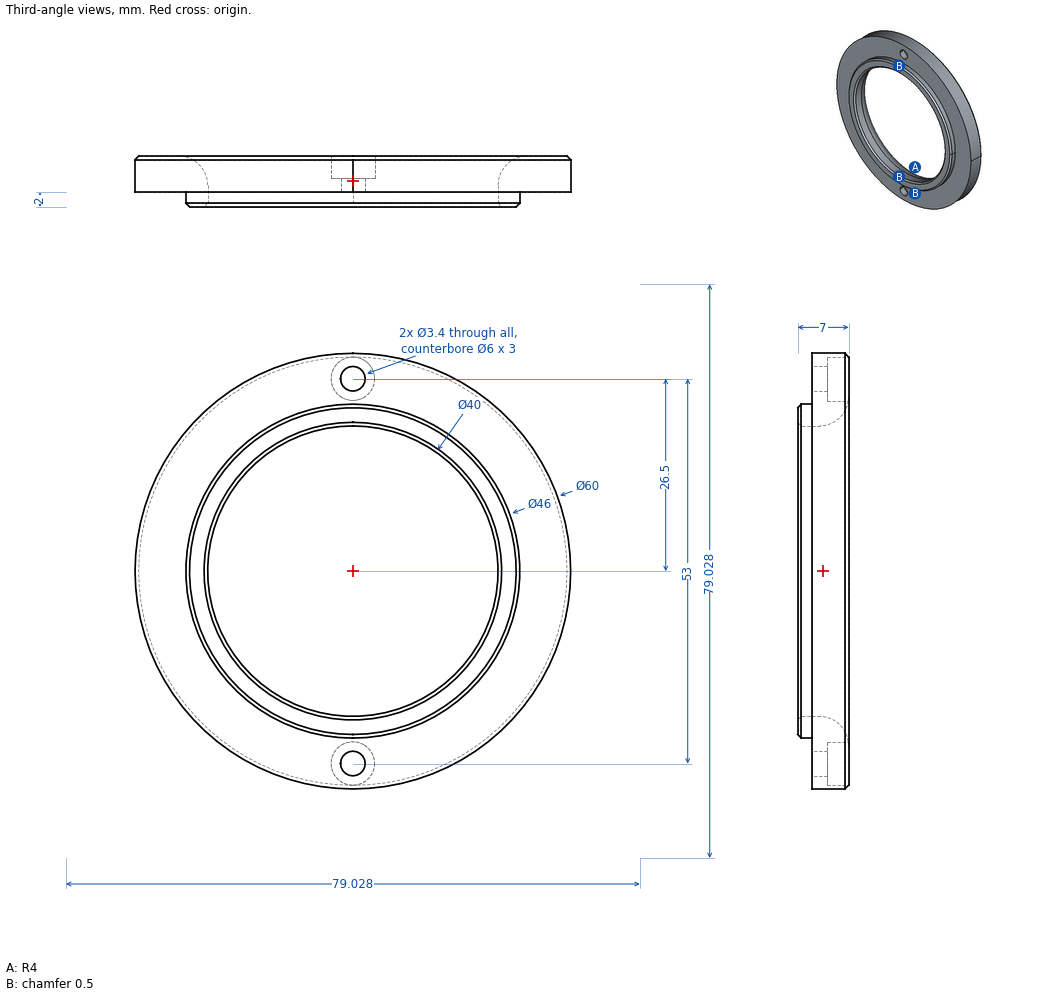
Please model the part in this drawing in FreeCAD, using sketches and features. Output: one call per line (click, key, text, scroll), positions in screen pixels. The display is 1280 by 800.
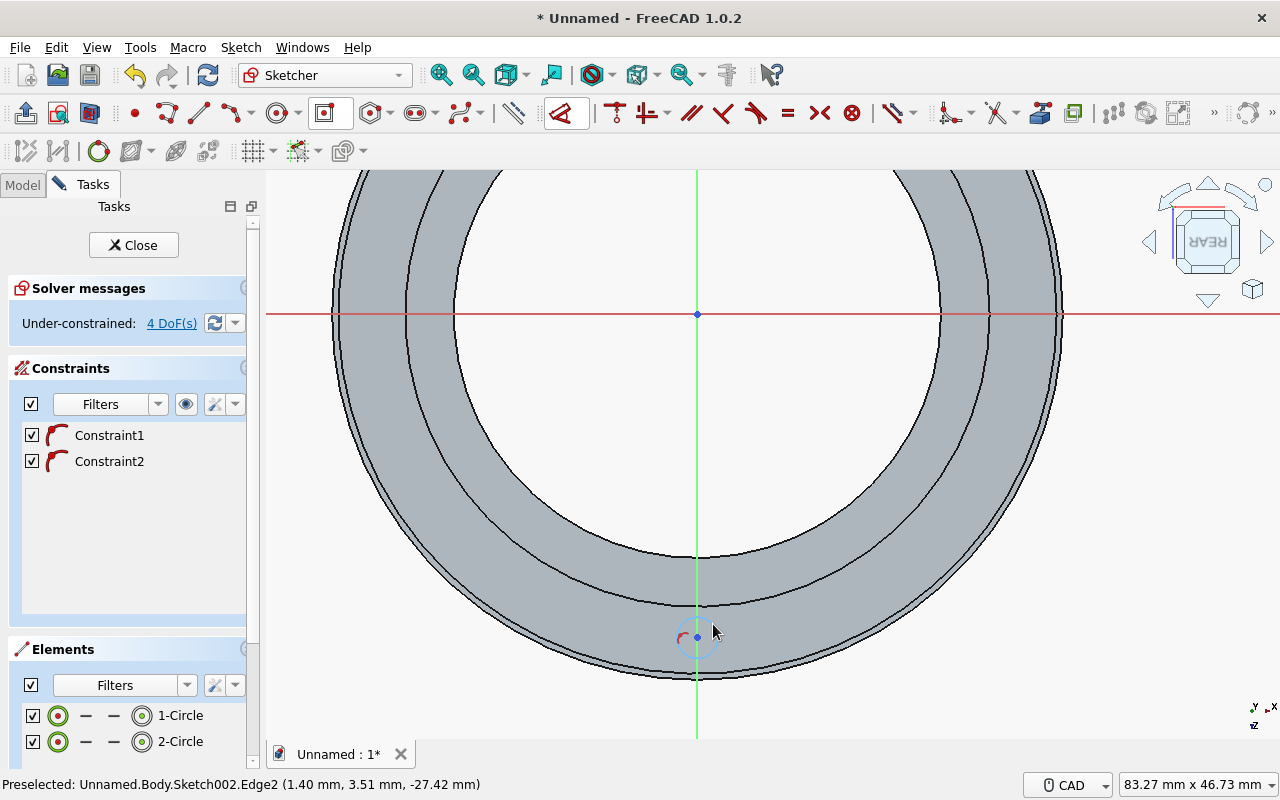
click(712, 623)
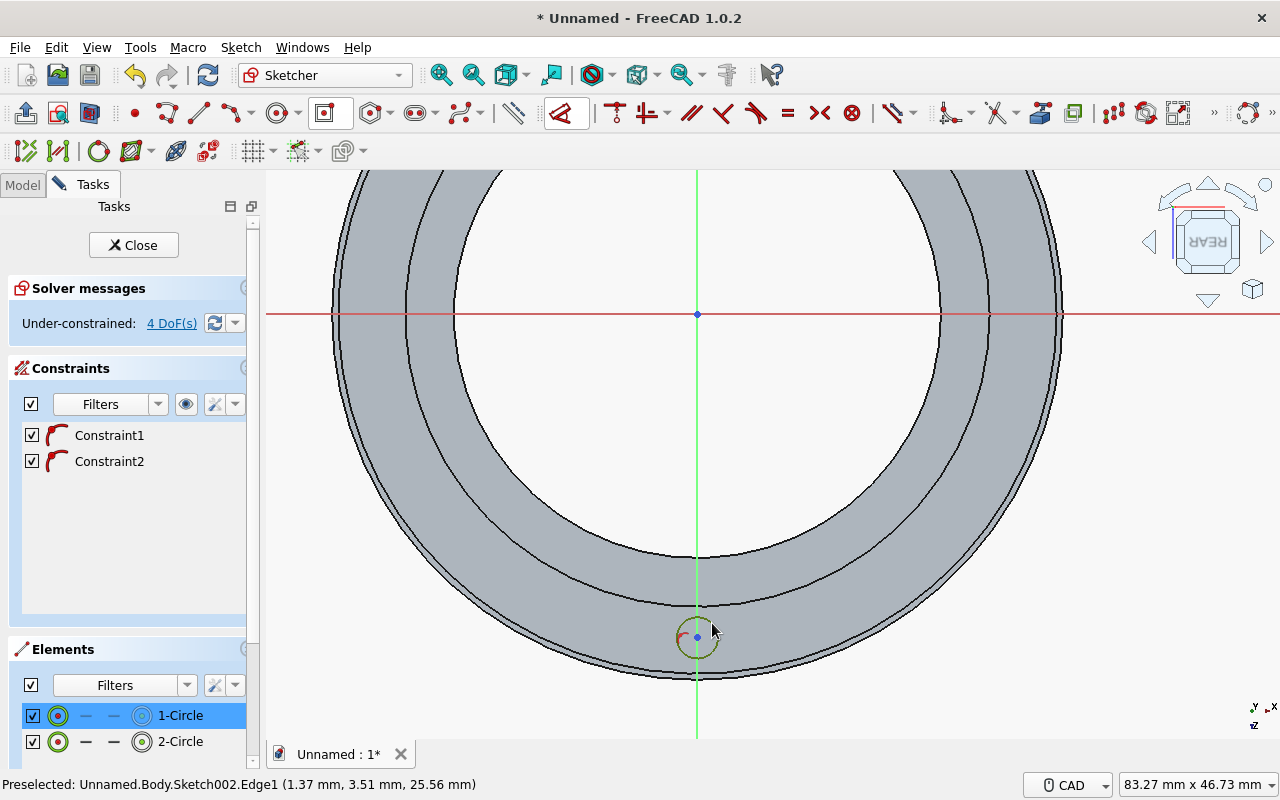
scroll(713, 625, down, 3)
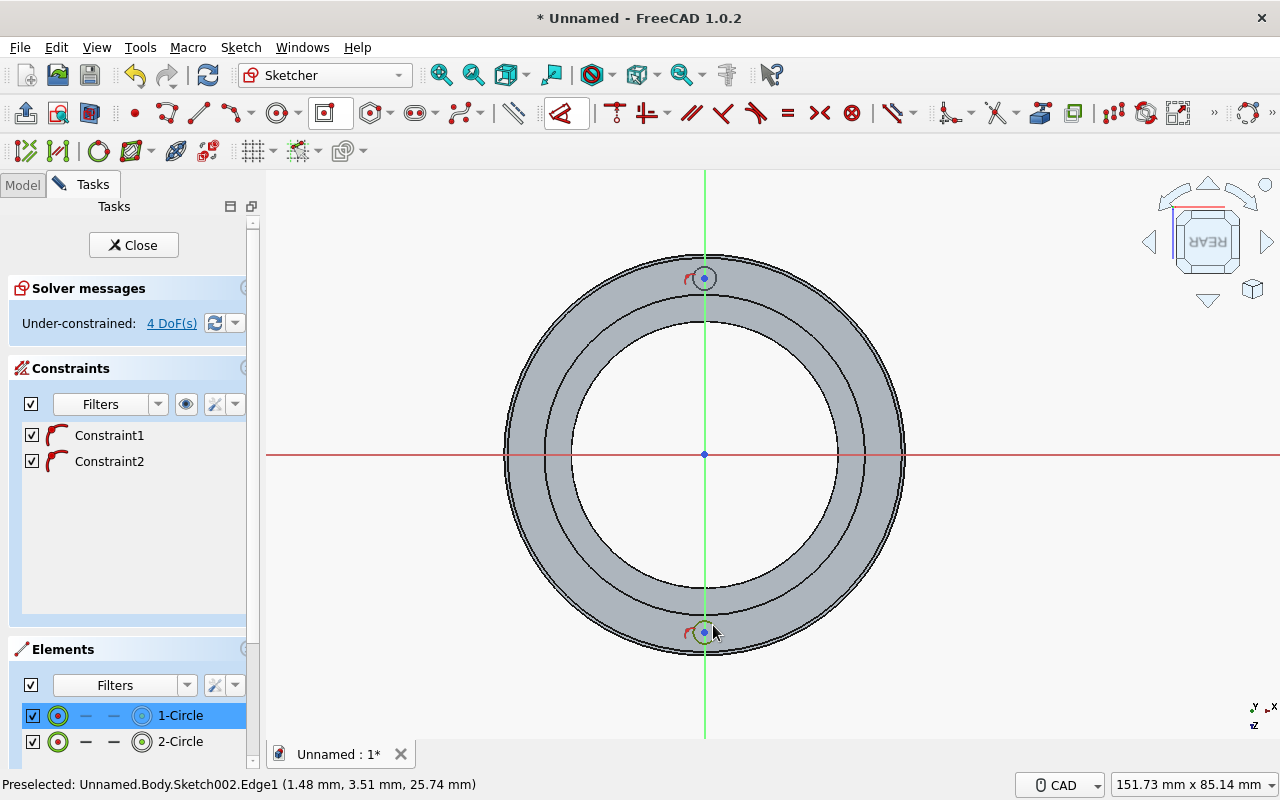
scroll(713, 270, up, 3)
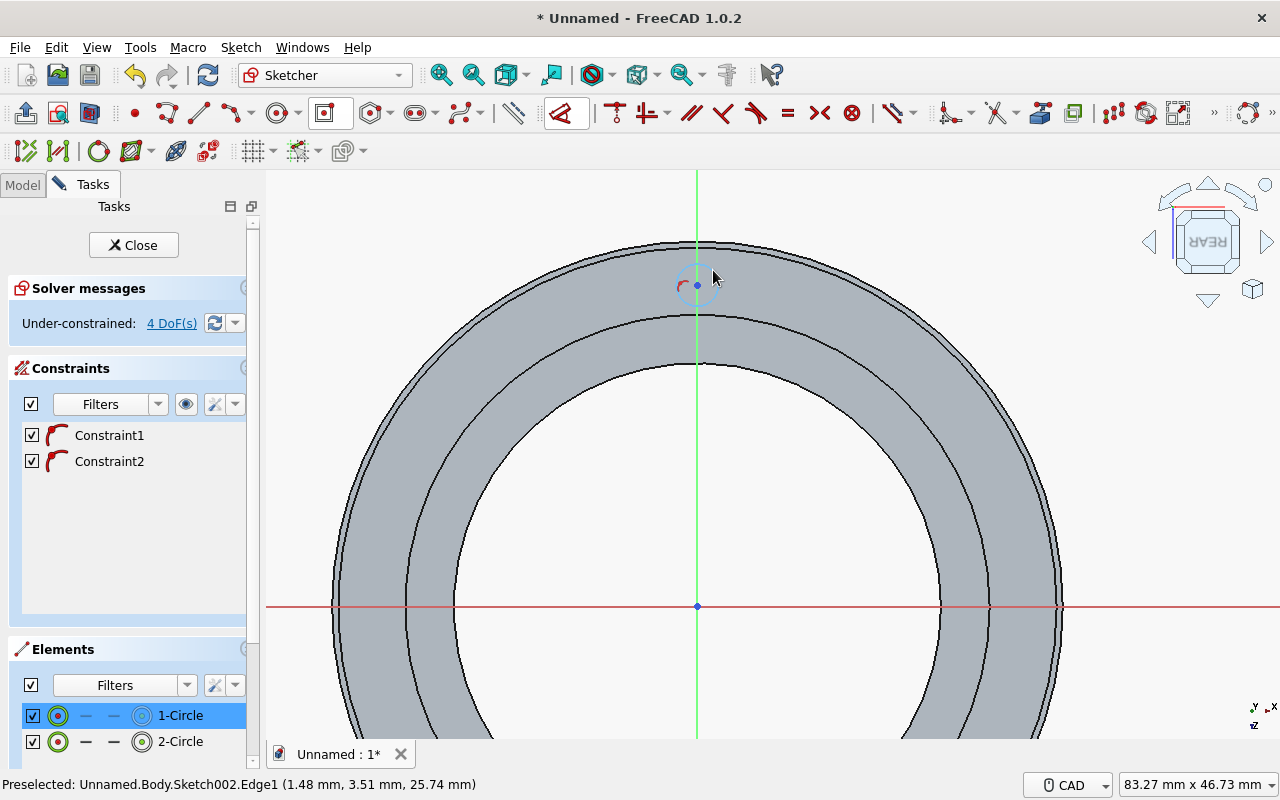
click(712, 270)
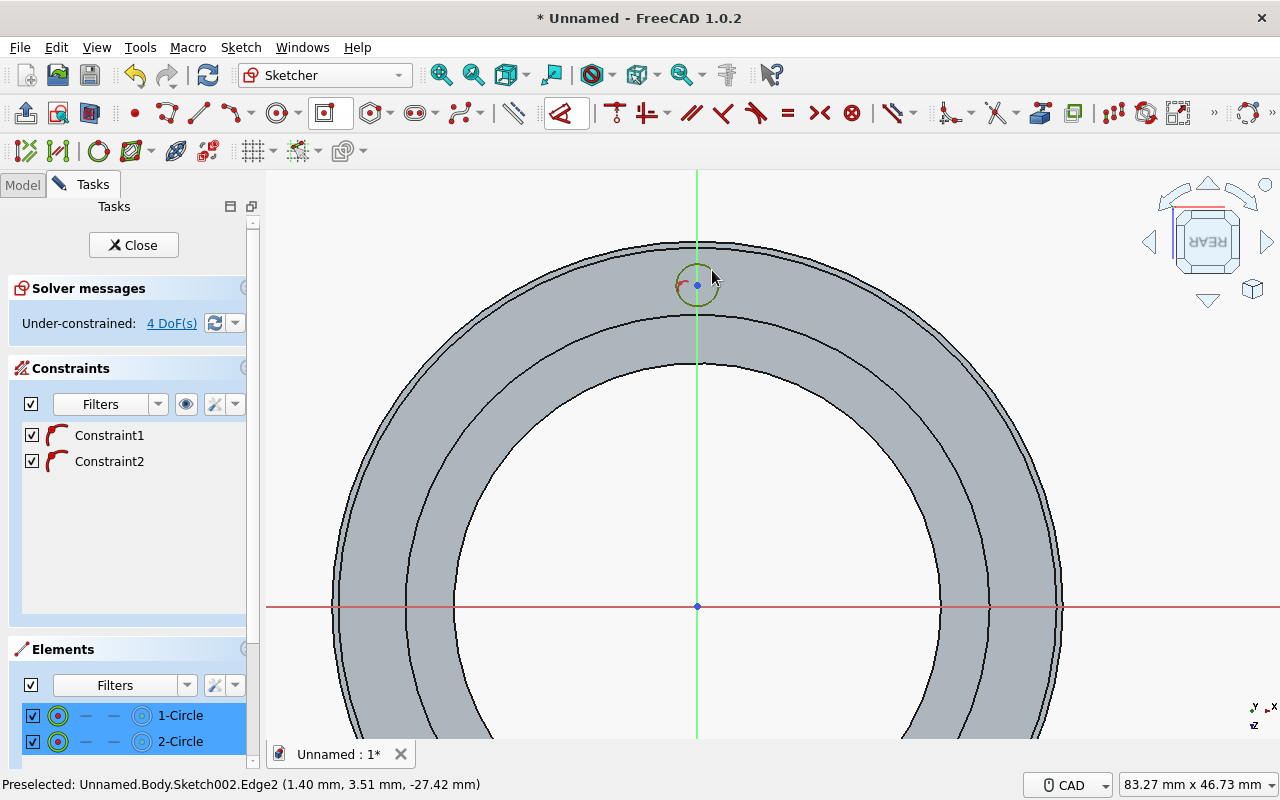
click(788, 114)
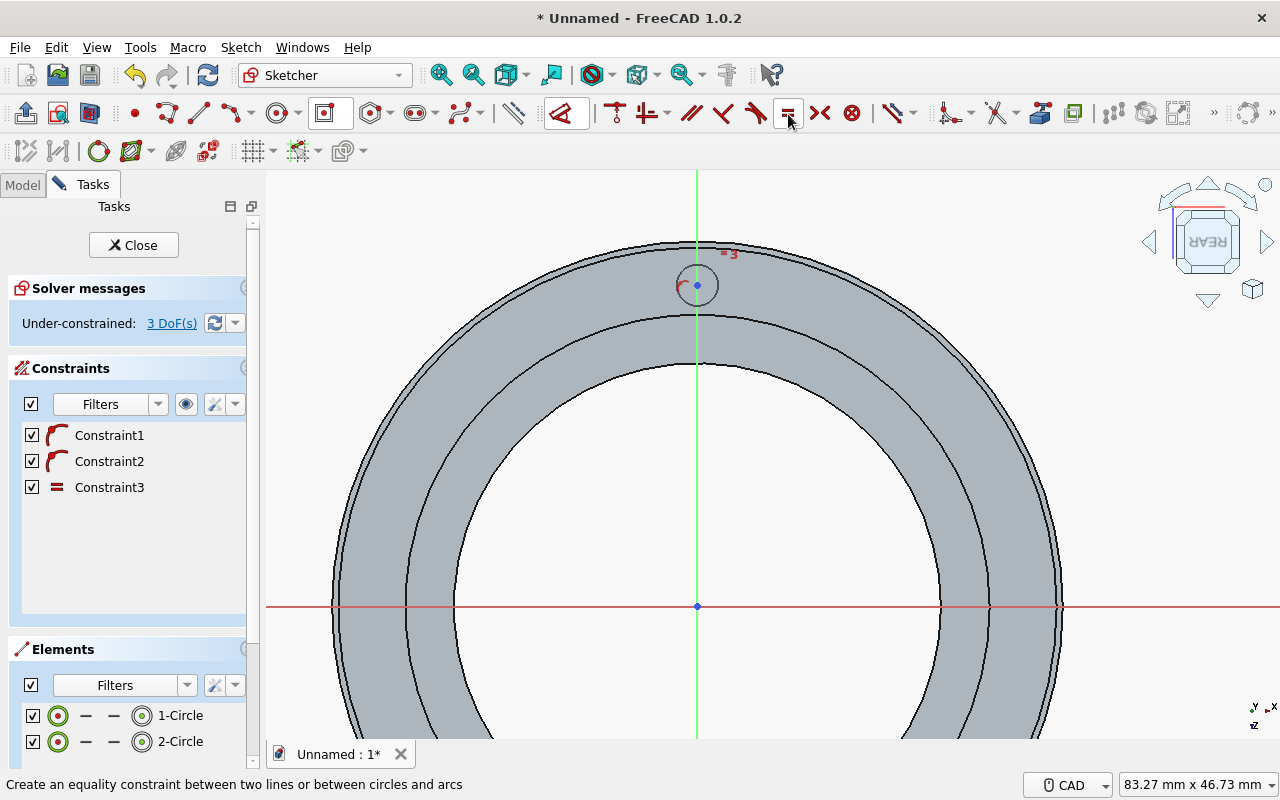
scroll(713, 269, down, 3)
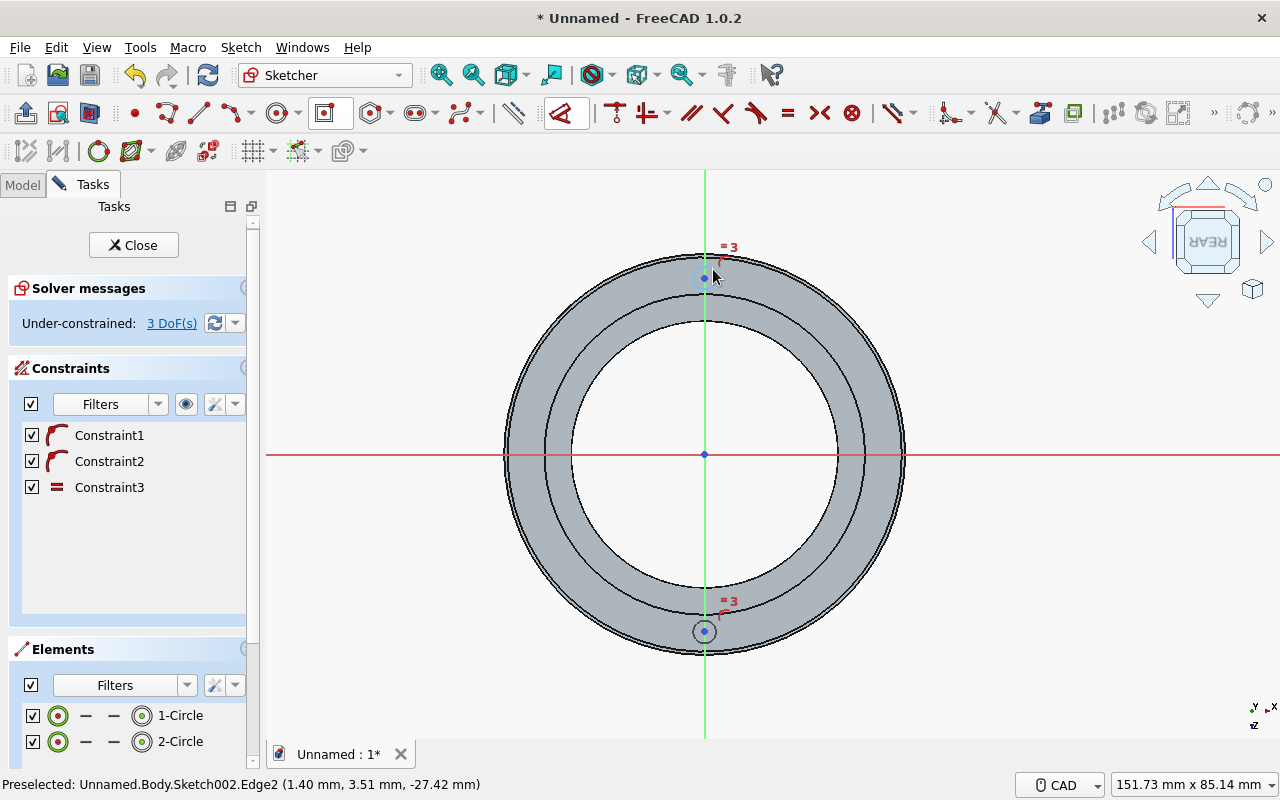
scroll(713, 624, up, 3)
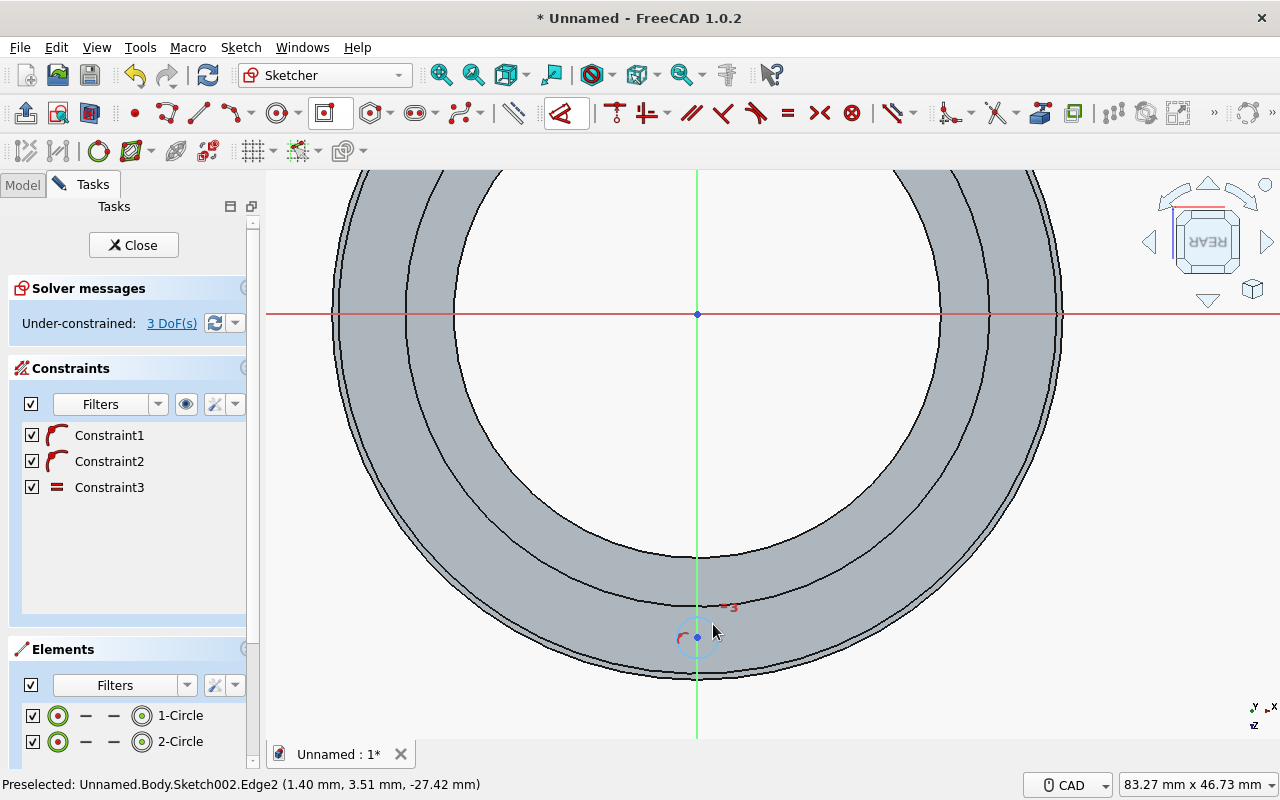
click(712, 623)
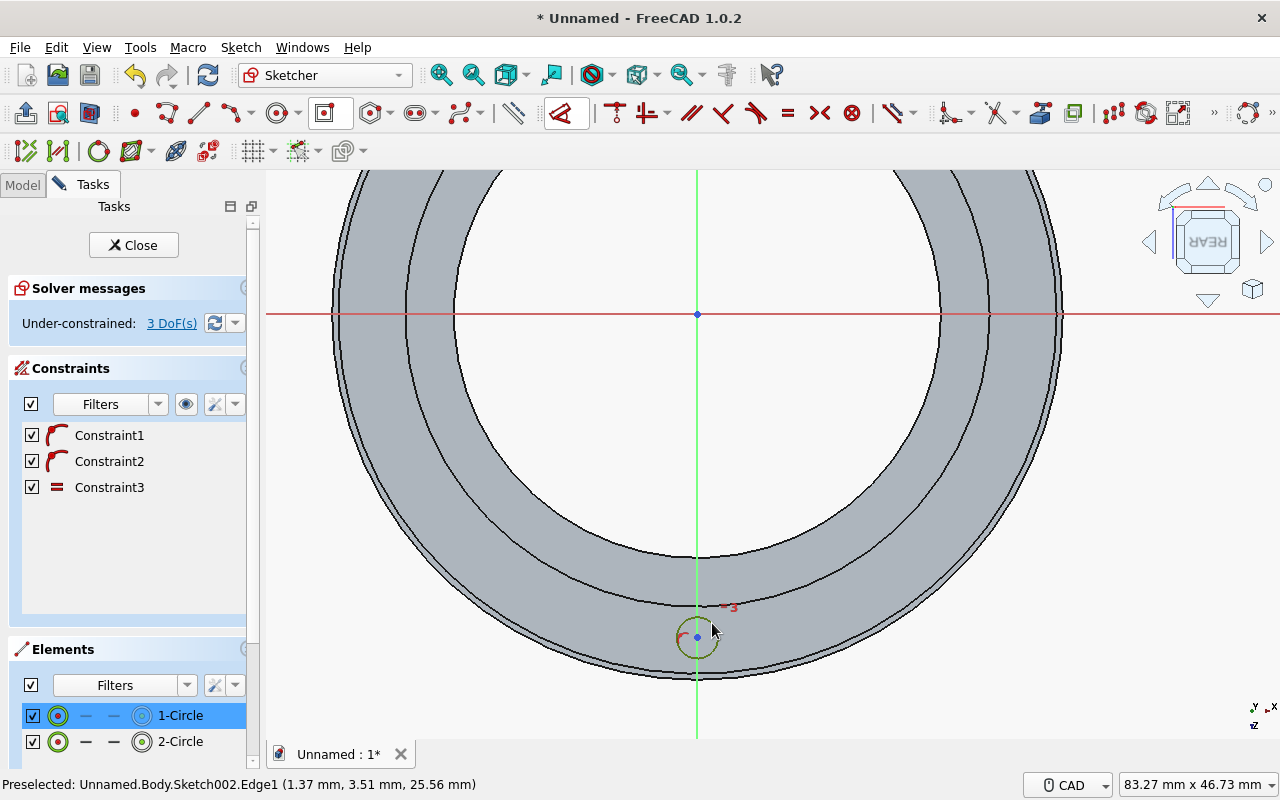
key(k)
key(o)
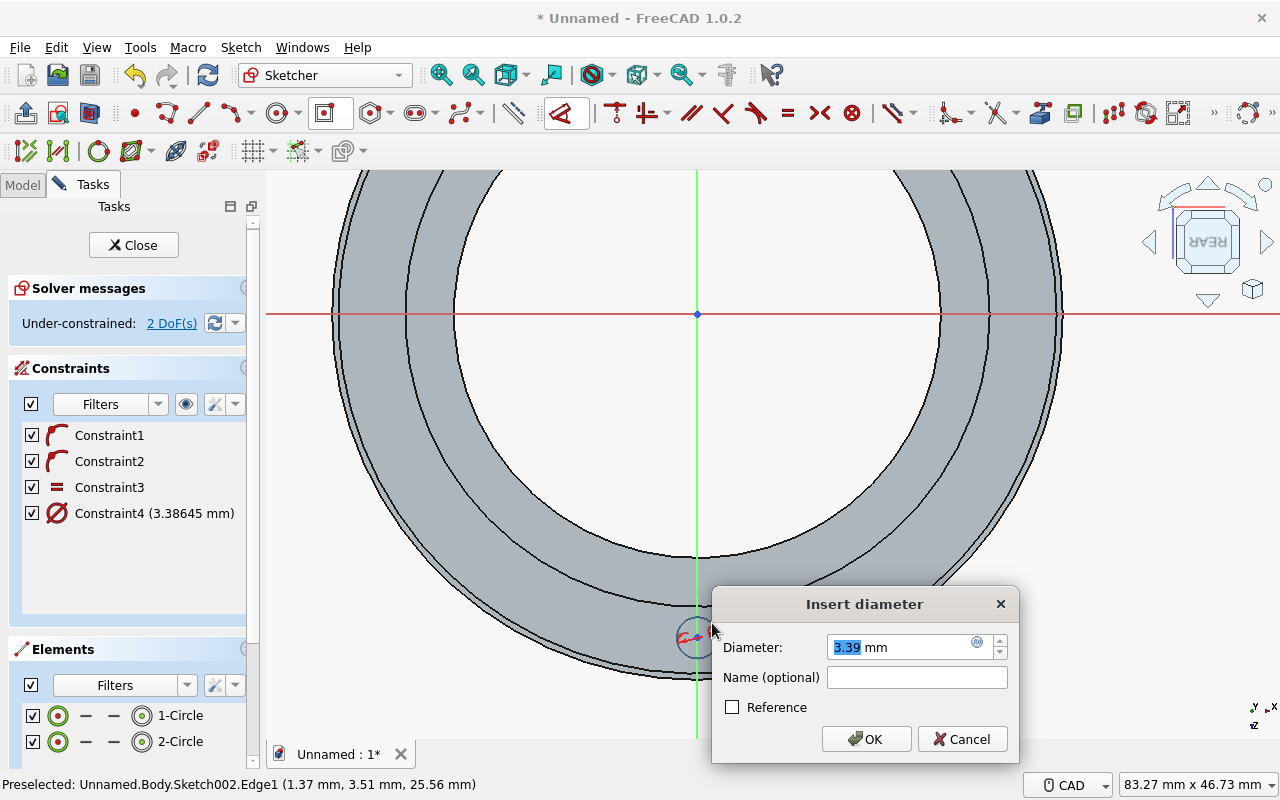
text(3.4)
key(Return)